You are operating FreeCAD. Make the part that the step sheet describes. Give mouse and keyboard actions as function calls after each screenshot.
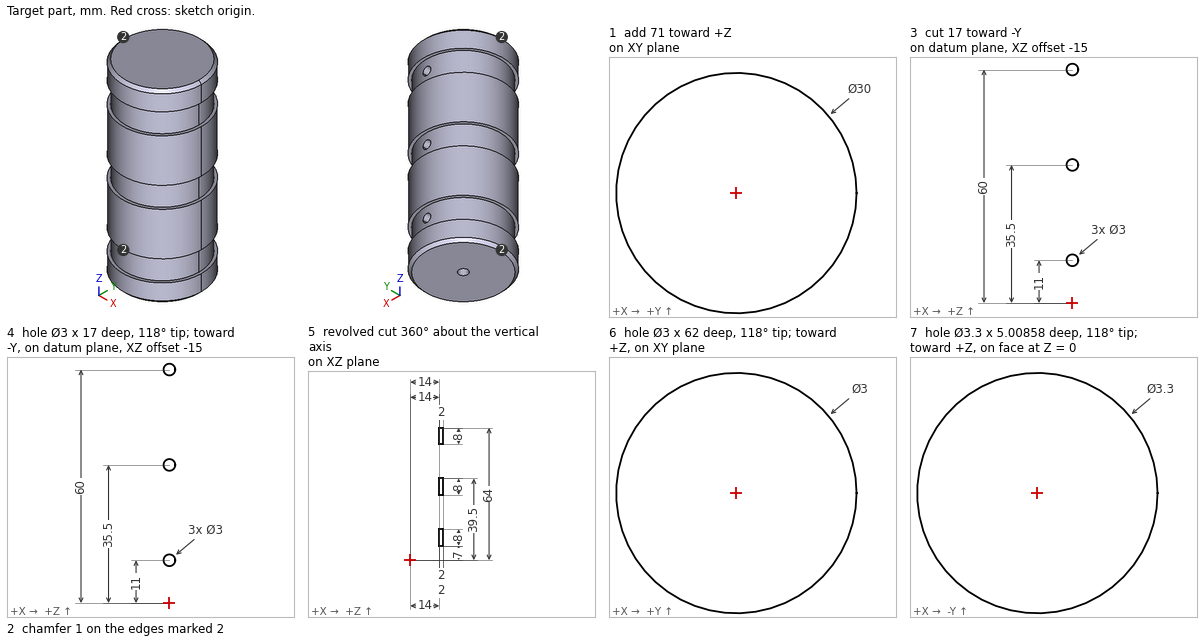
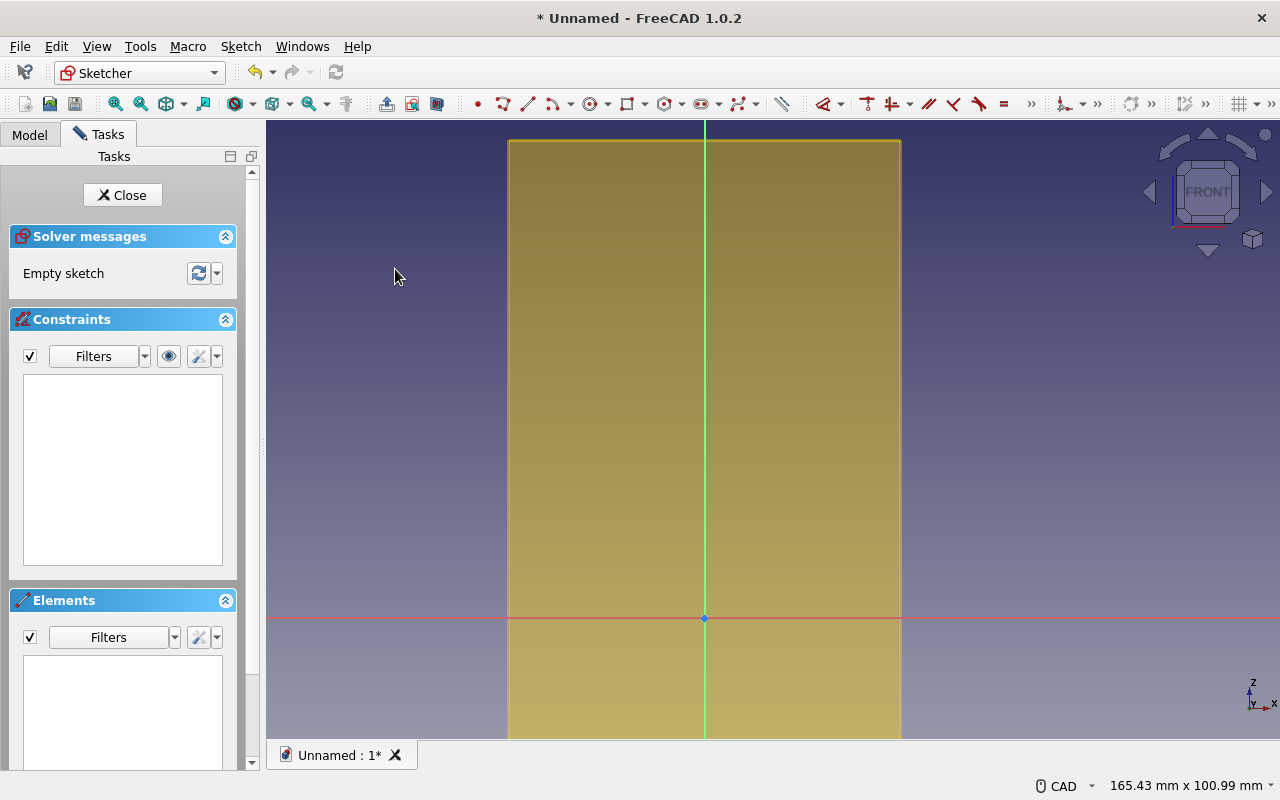
click(590, 104)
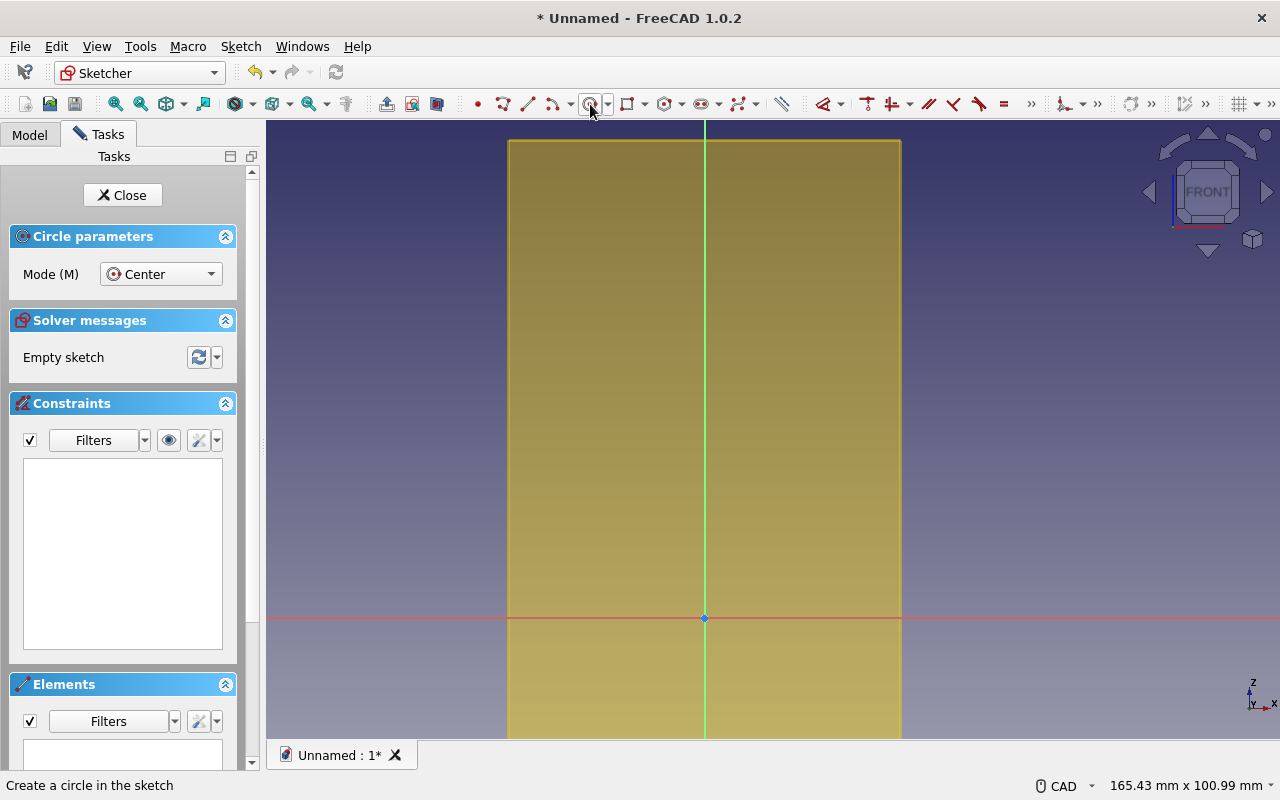
scroll(705, 551, up, 5)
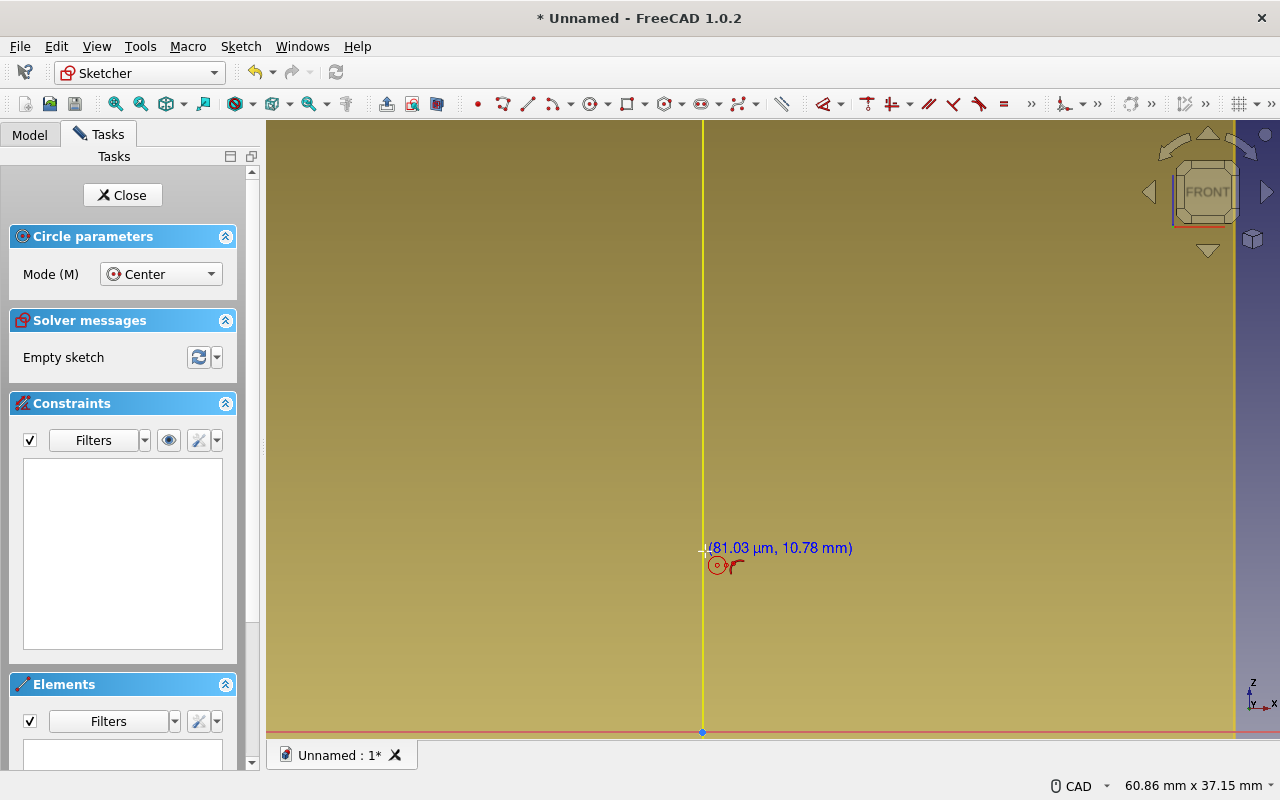
click(703, 549)
move(721, 531)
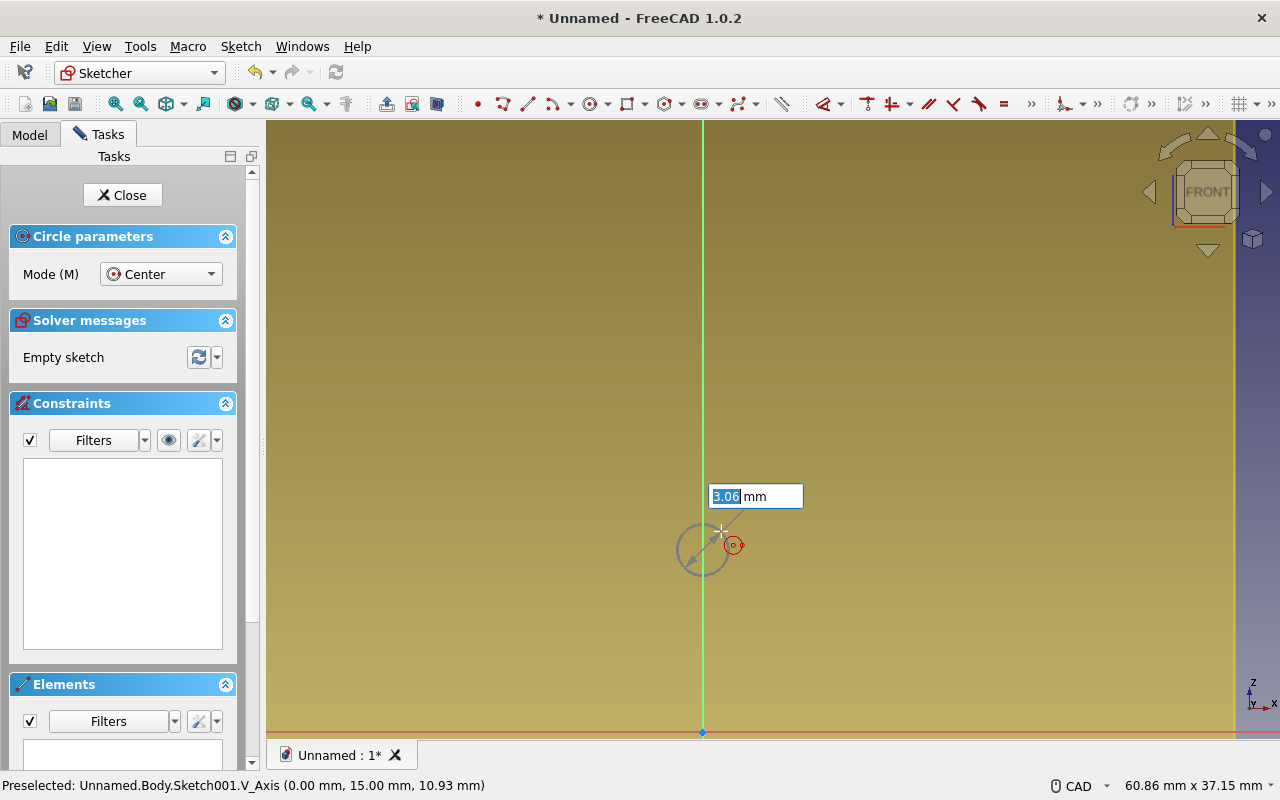
text(3)
key(Return)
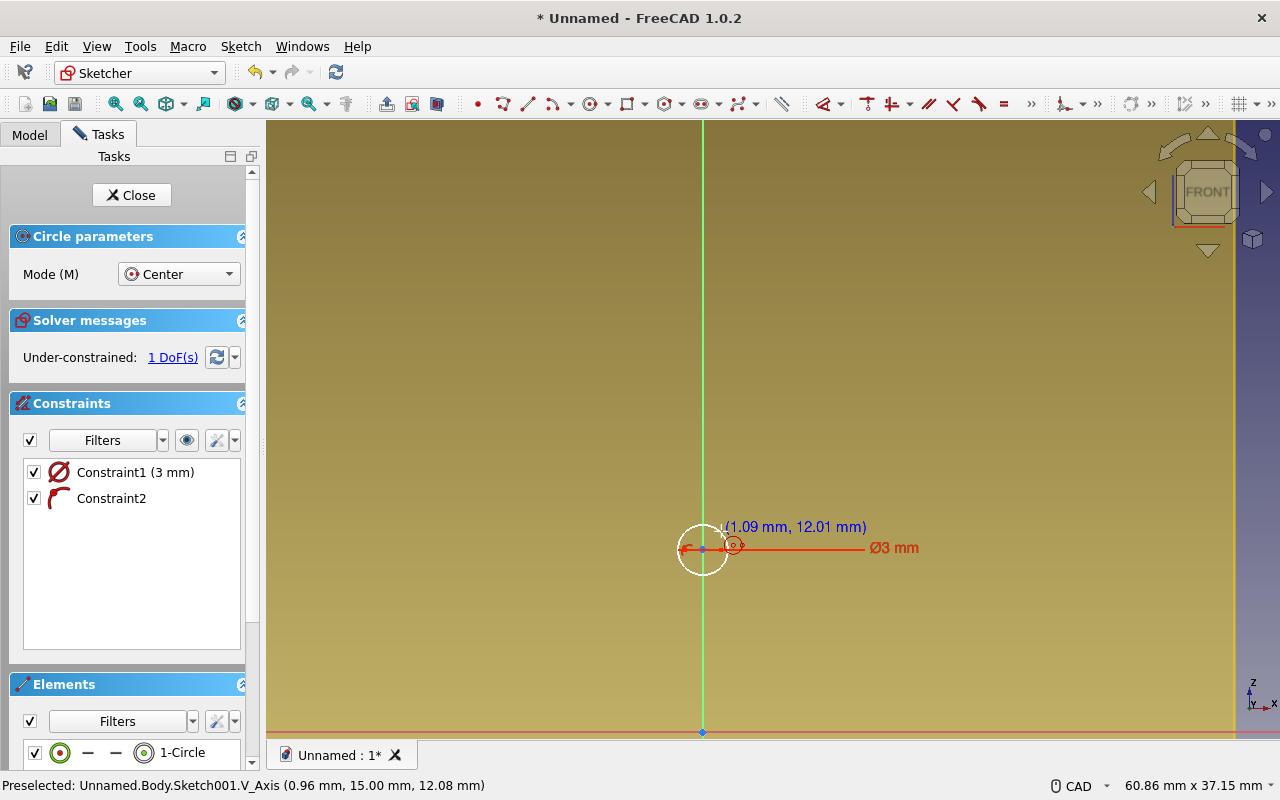
scroll(705, 552, down, 5)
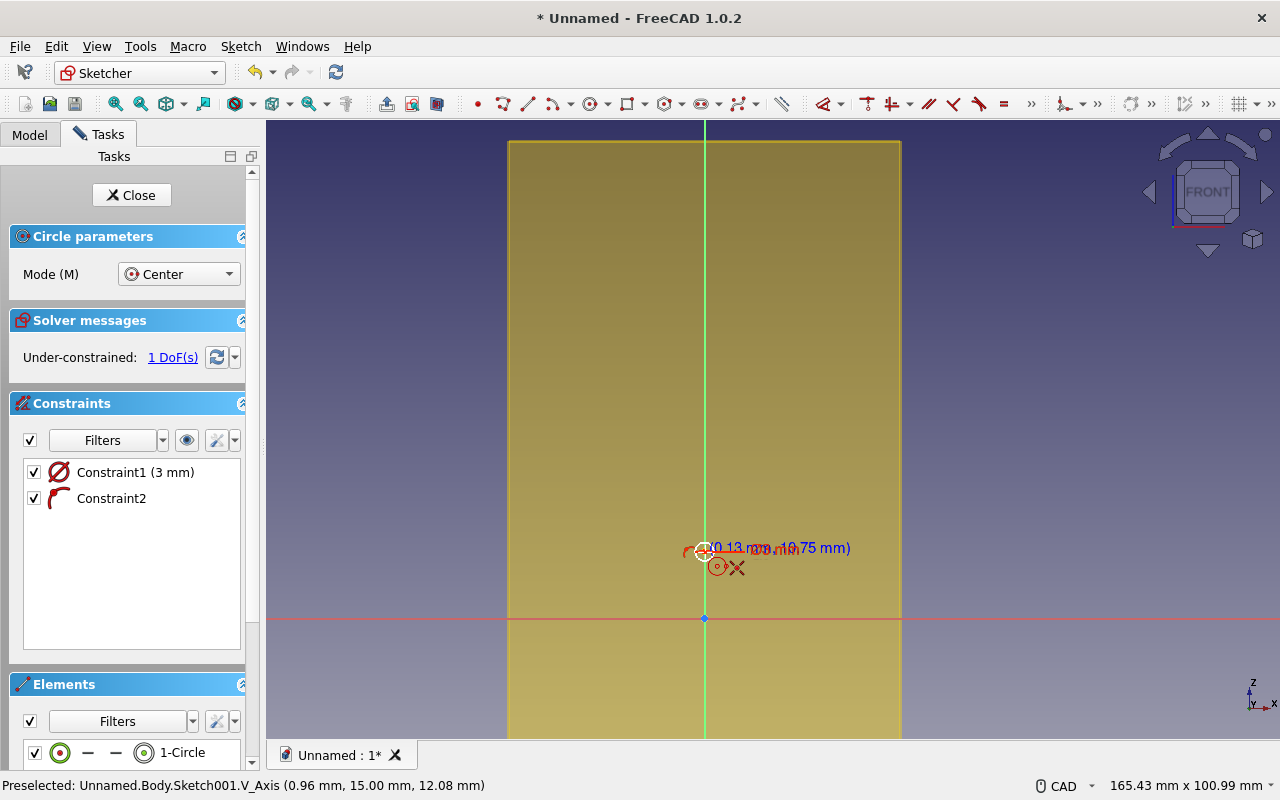
scroll(705, 401, up, 5)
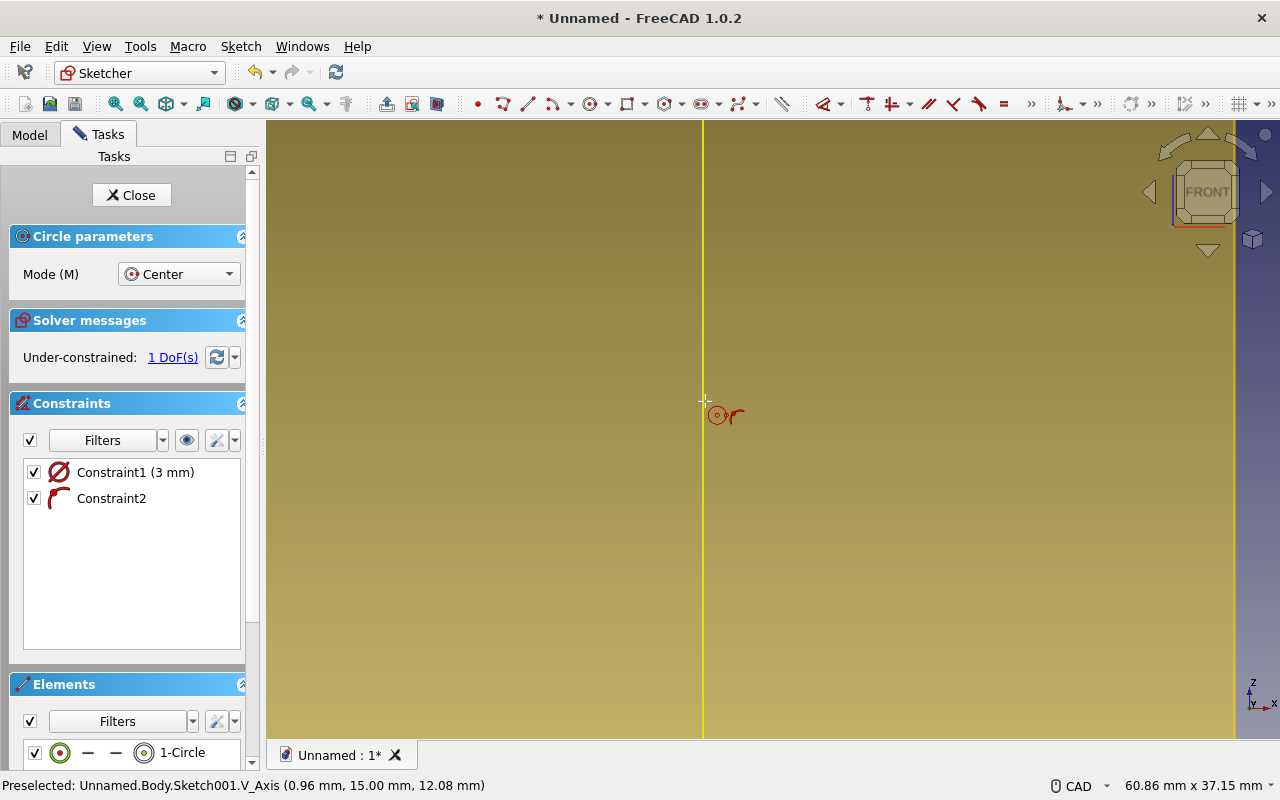
click(703, 400)
move(721, 383)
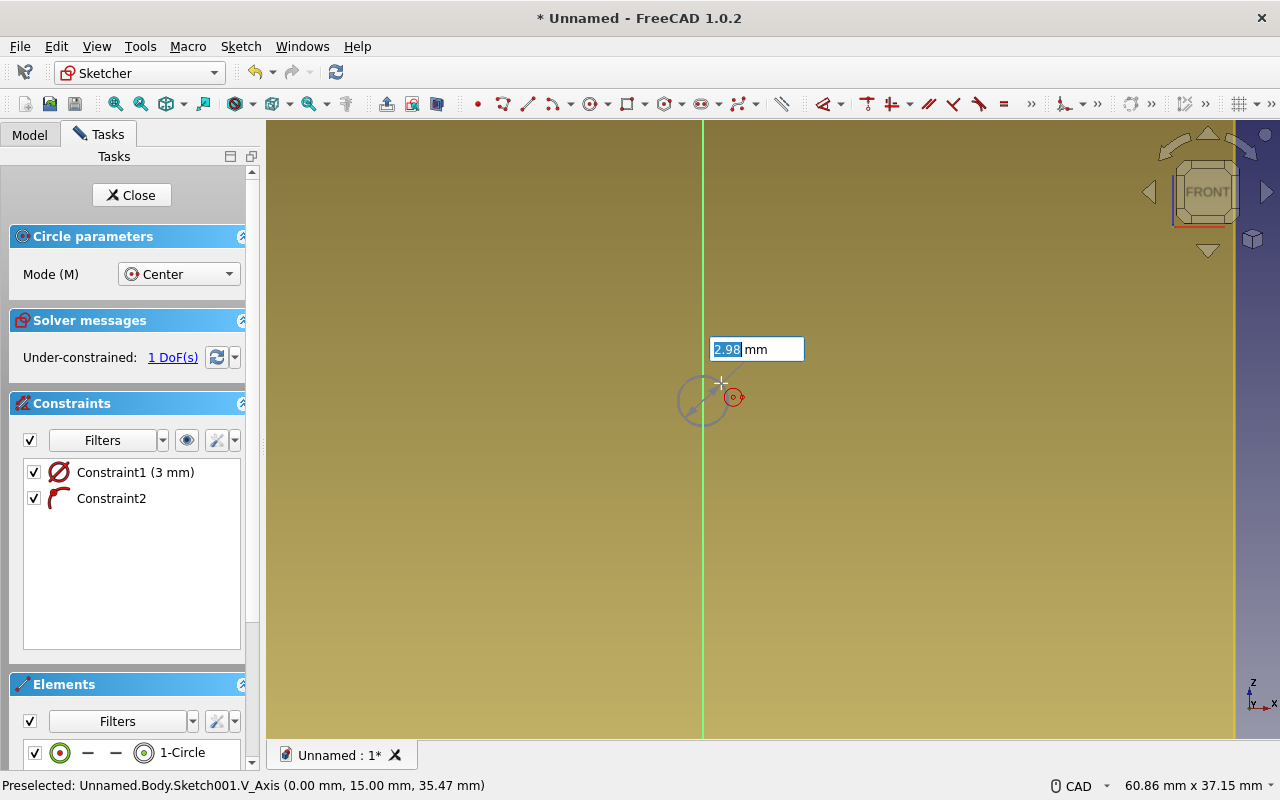
text(3)
key(Return)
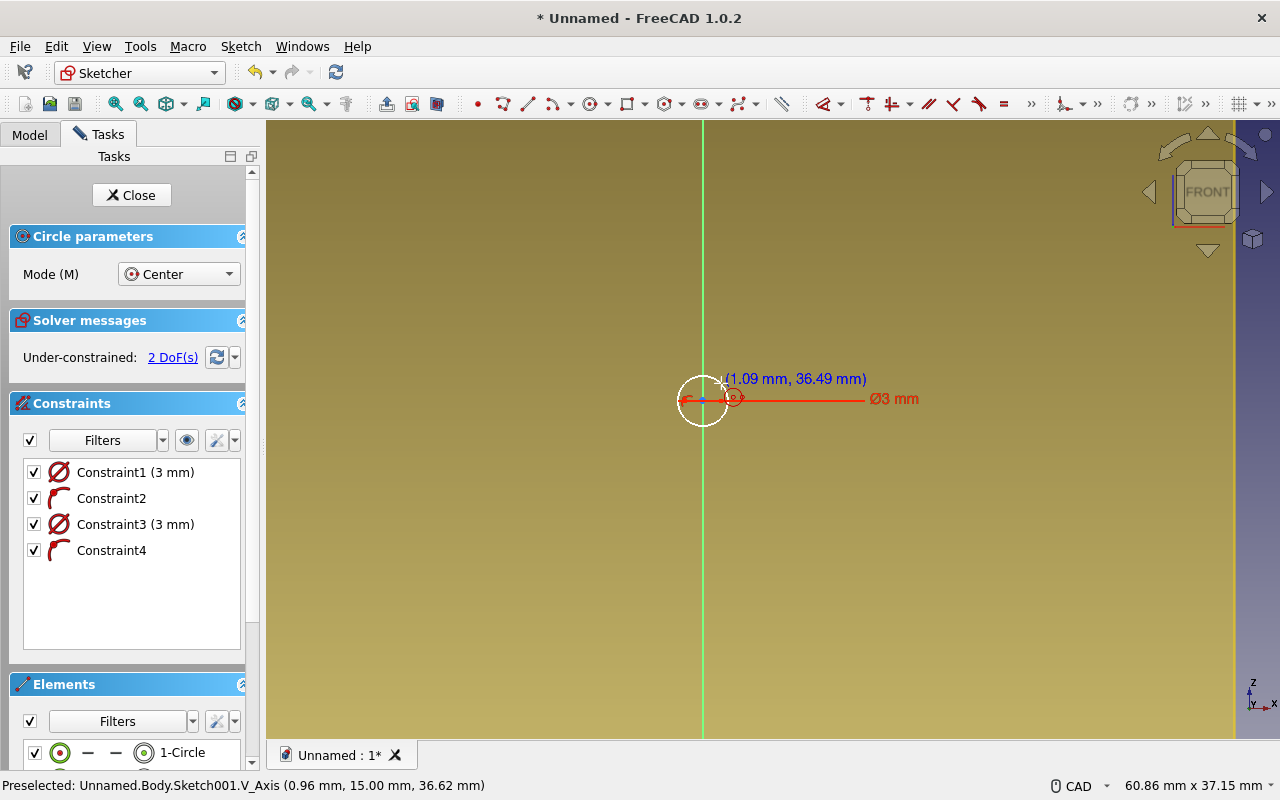
scroll(705, 400, down, 5)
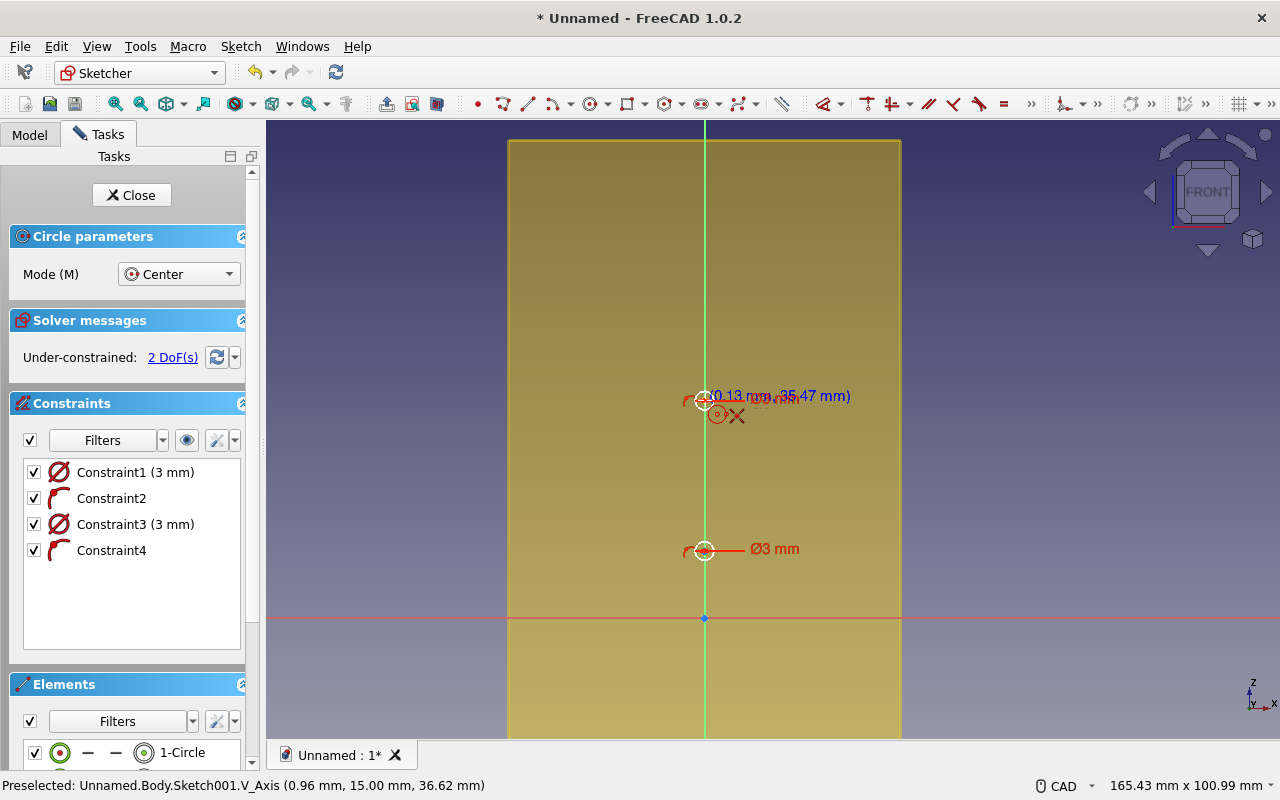
scroll(705, 250, up, 5)